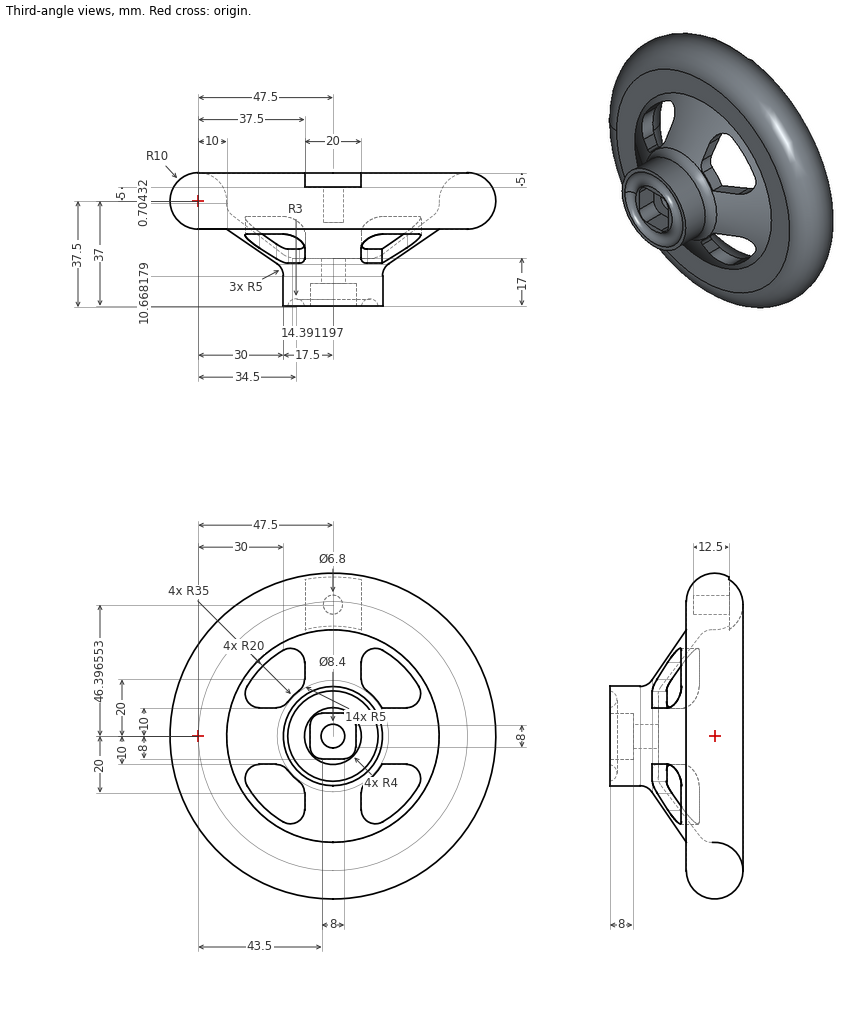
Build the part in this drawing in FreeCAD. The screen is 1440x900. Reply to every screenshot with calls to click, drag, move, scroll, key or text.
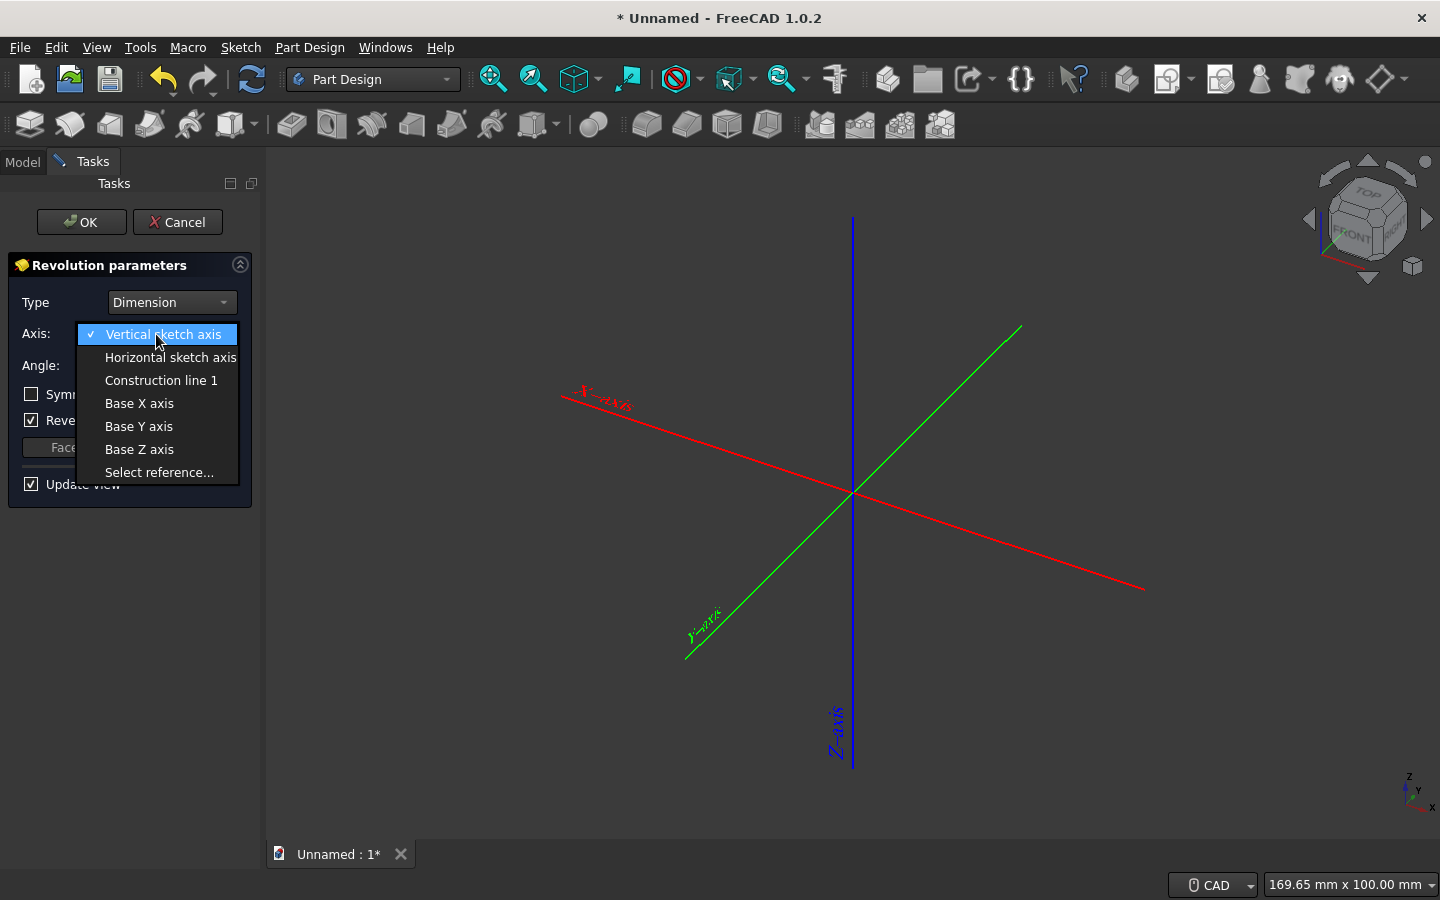
click(156, 380)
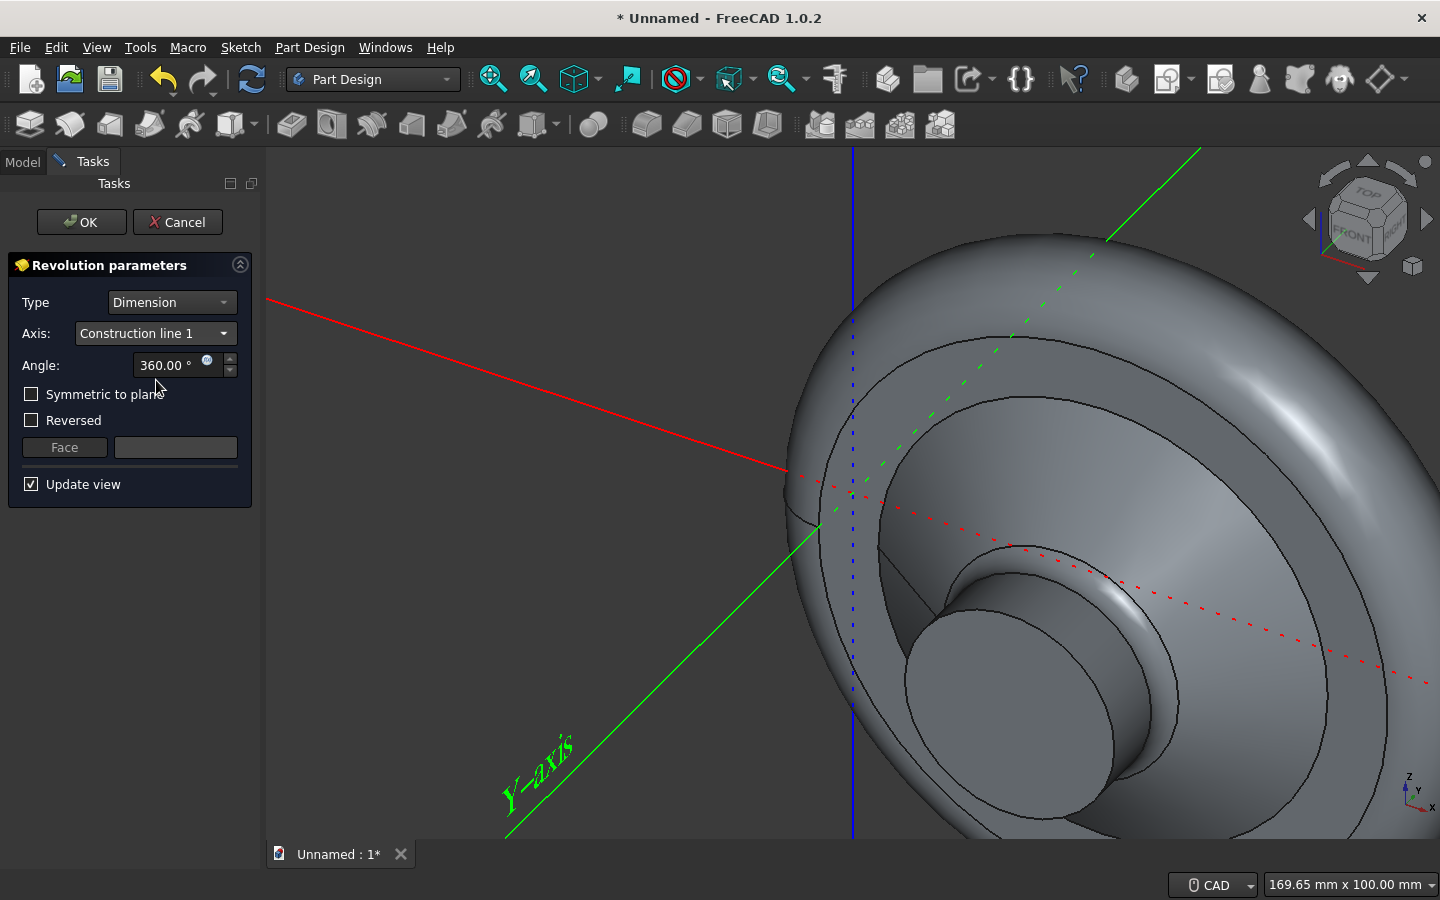
click(82, 222)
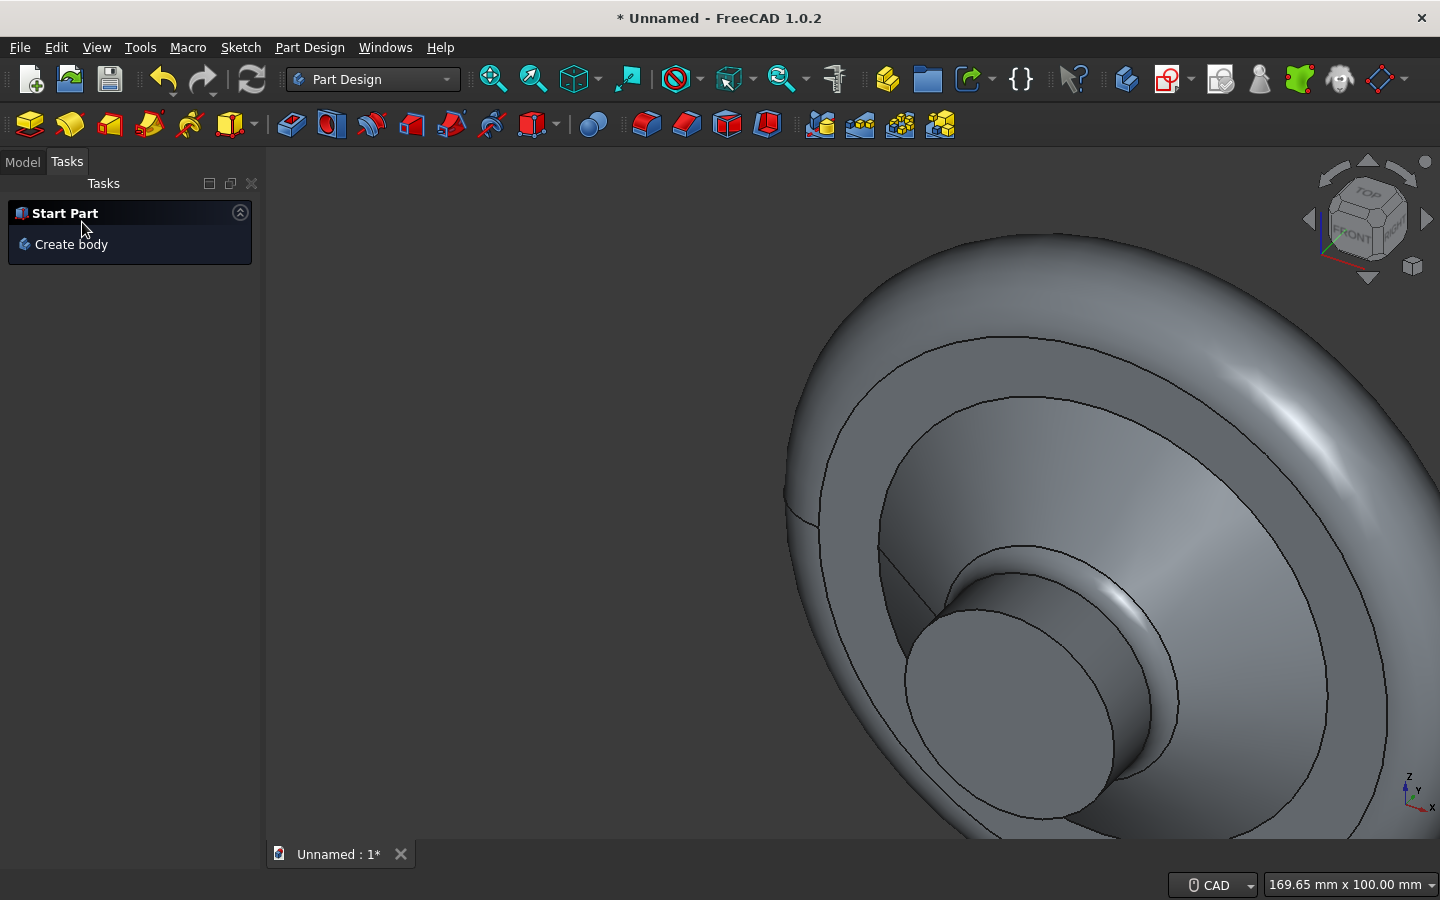
click(494, 80)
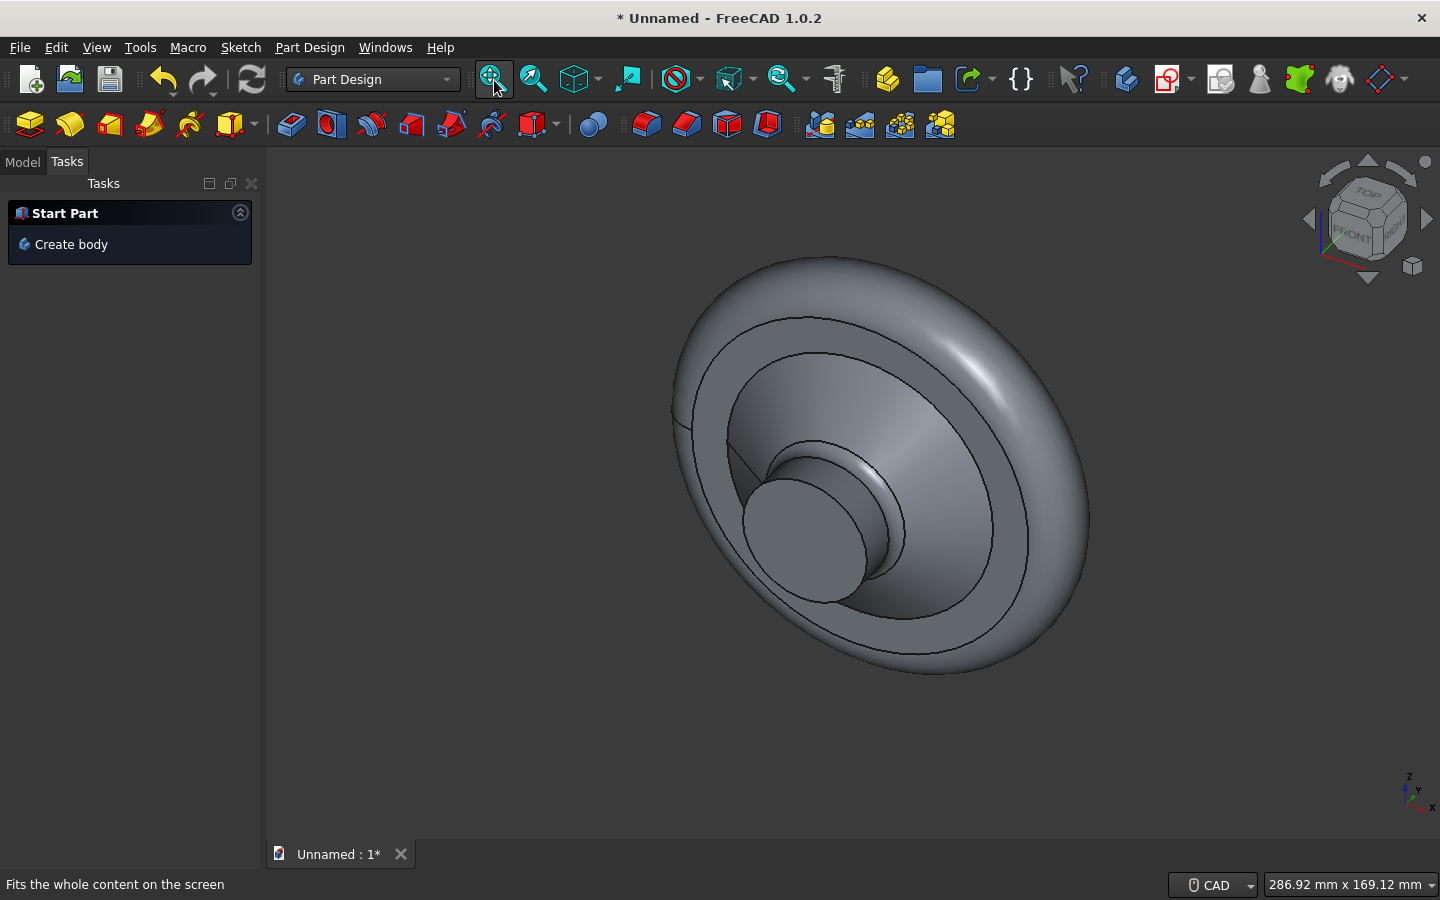
click(805, 540)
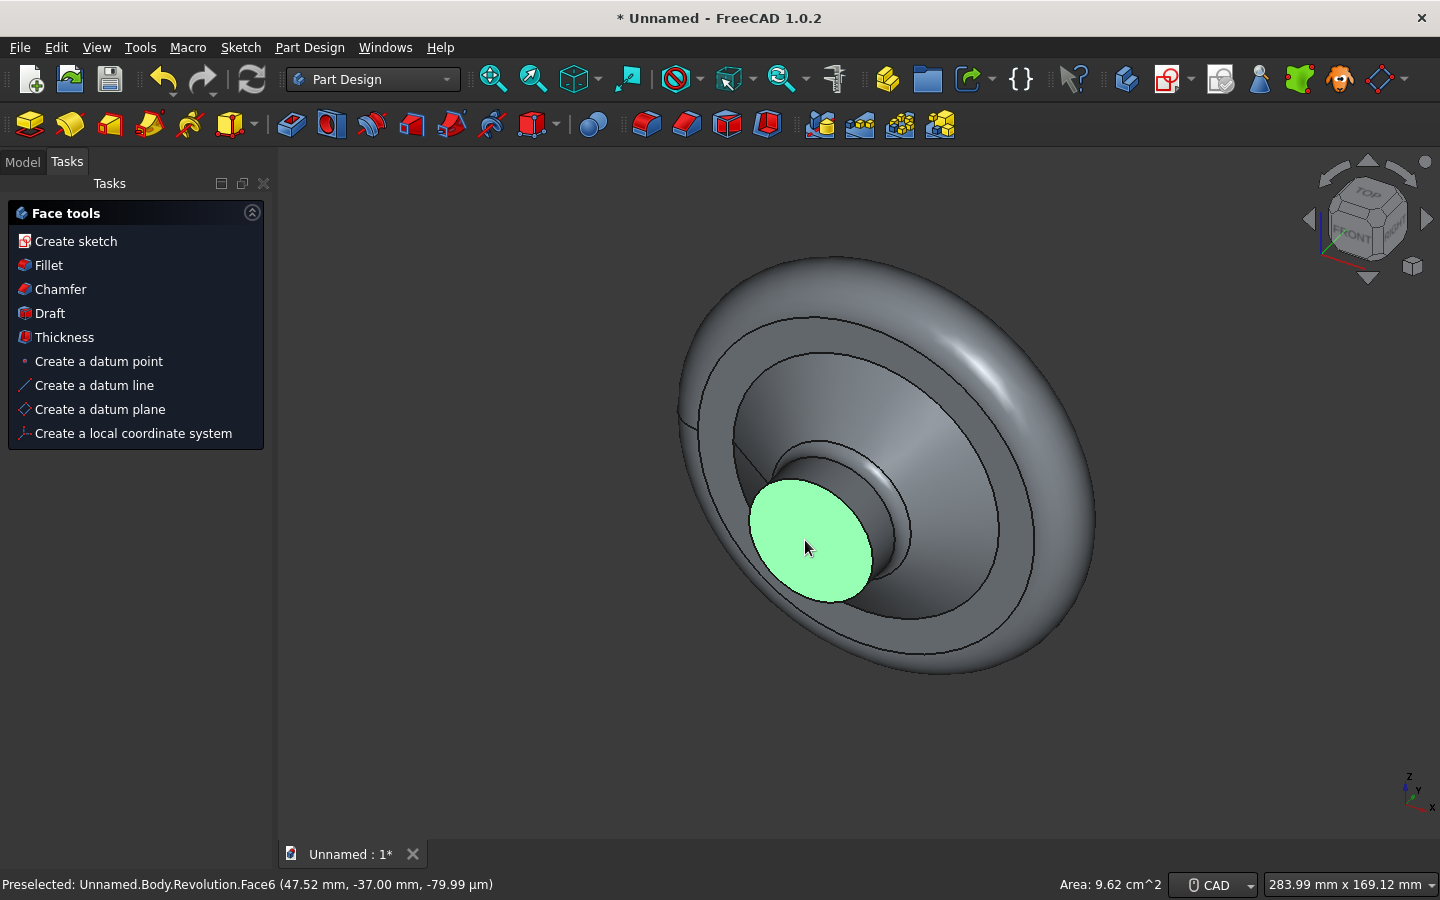
click(1168, 80)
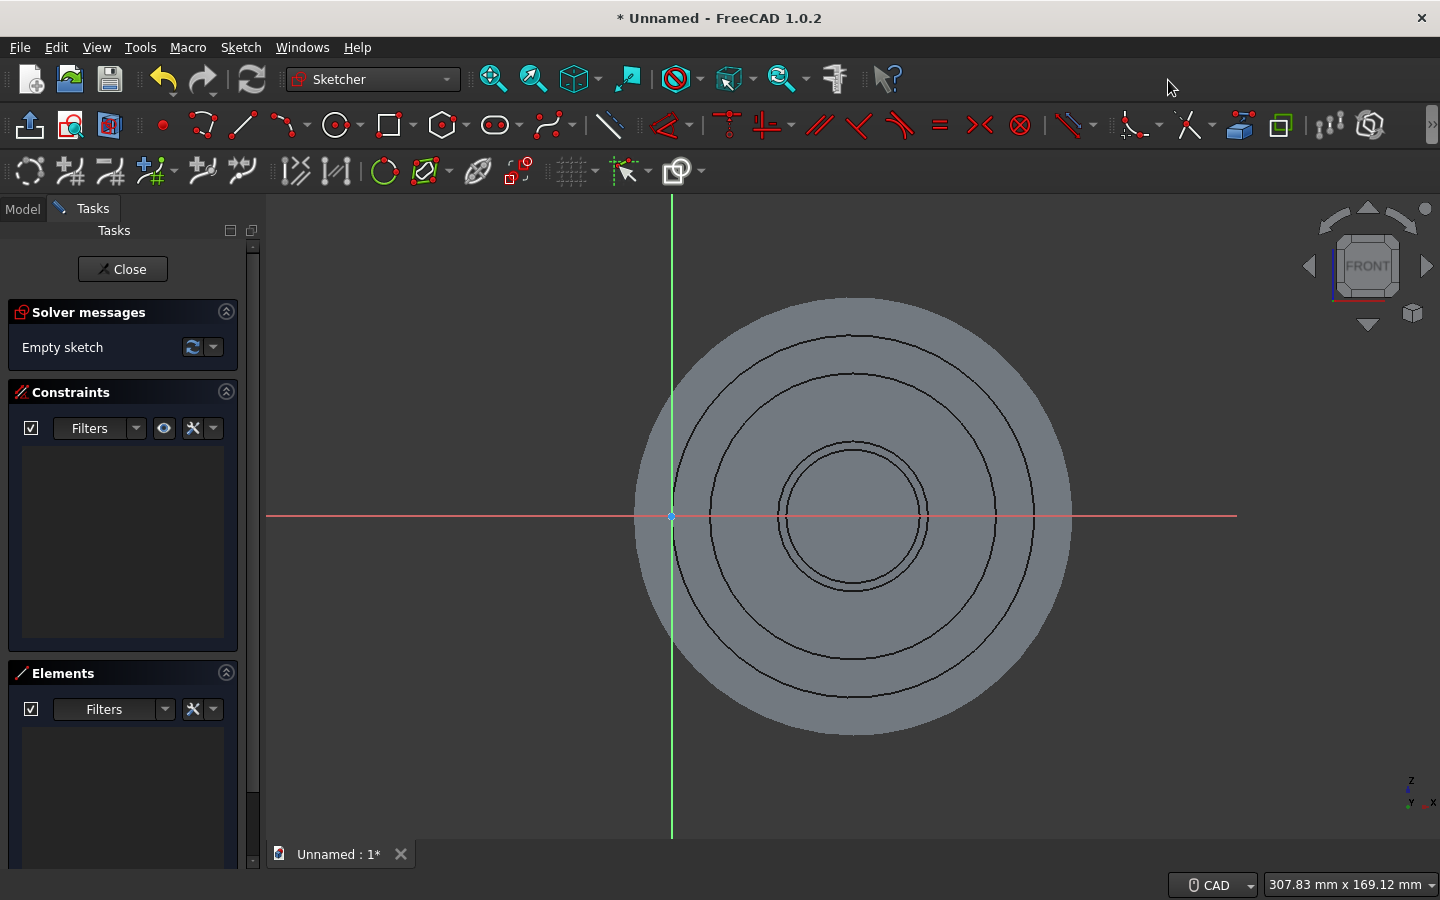
scroll(864, 516, up, 10)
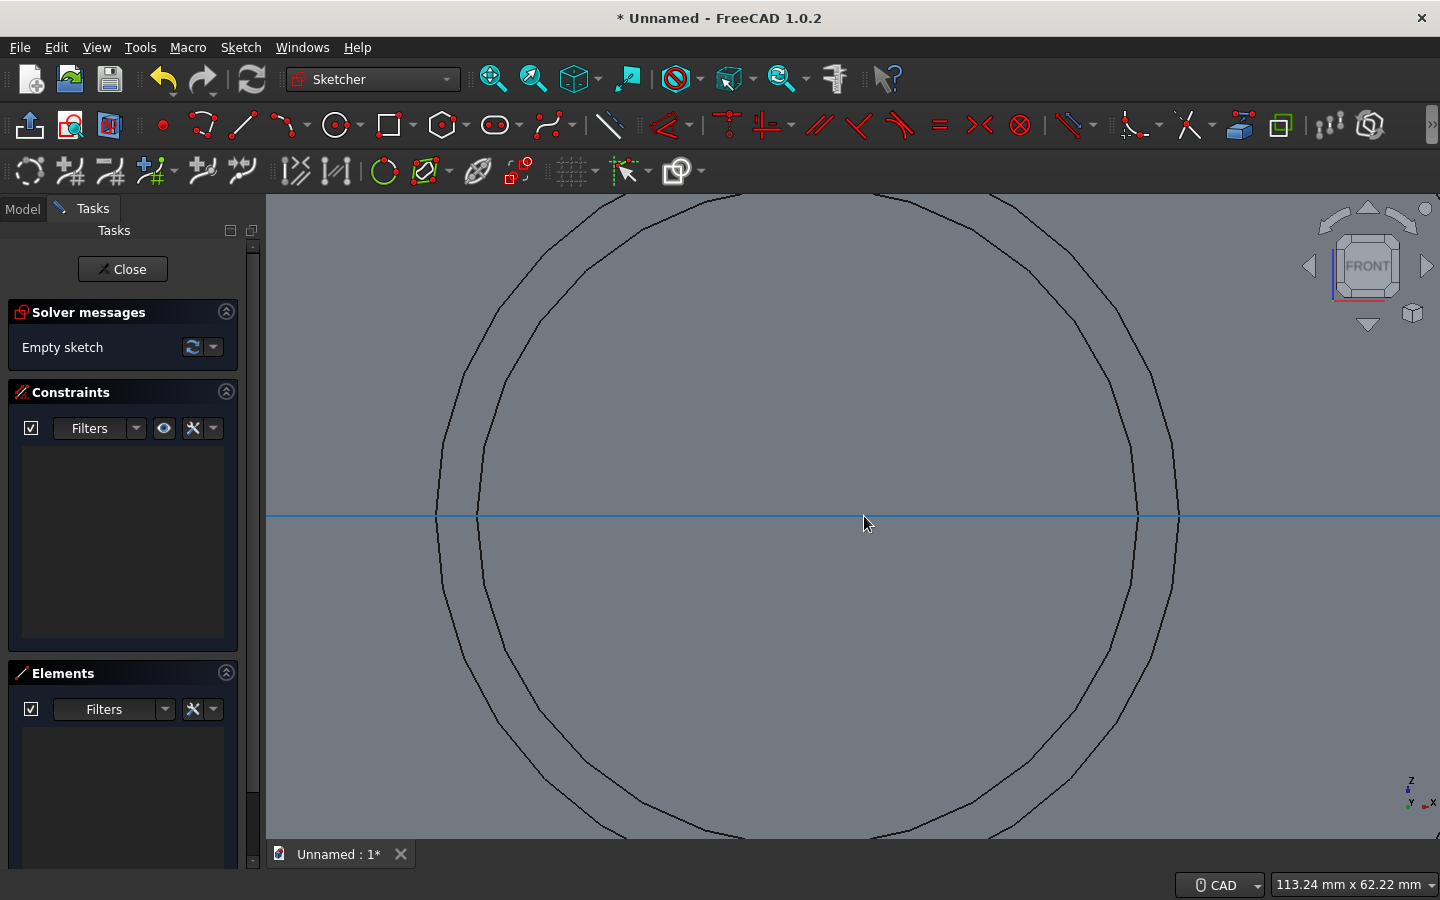
click(244, 126)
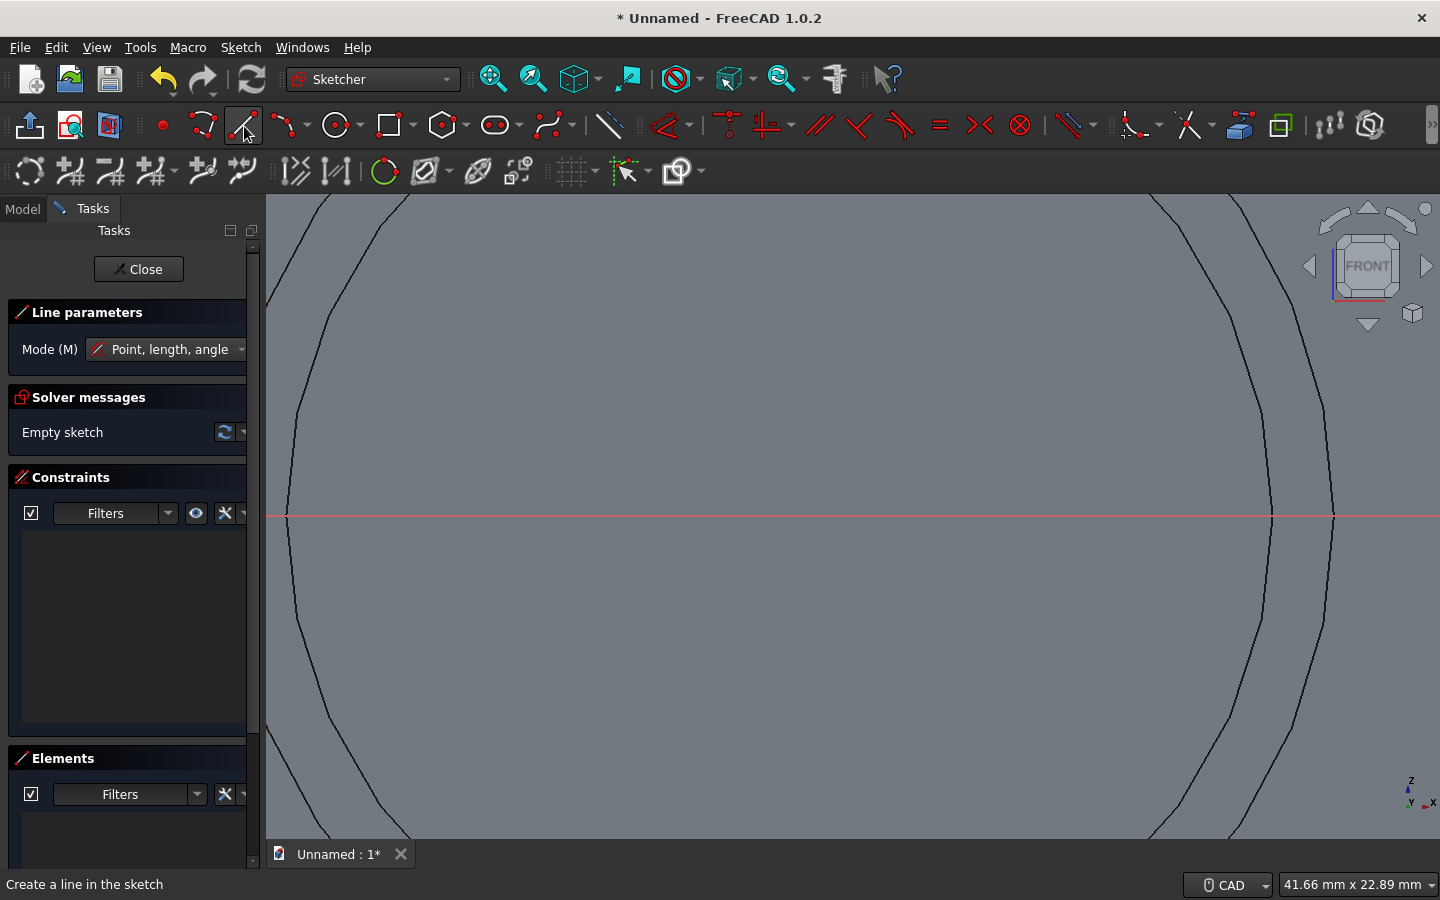
click(667, 742)
click(892, 742)